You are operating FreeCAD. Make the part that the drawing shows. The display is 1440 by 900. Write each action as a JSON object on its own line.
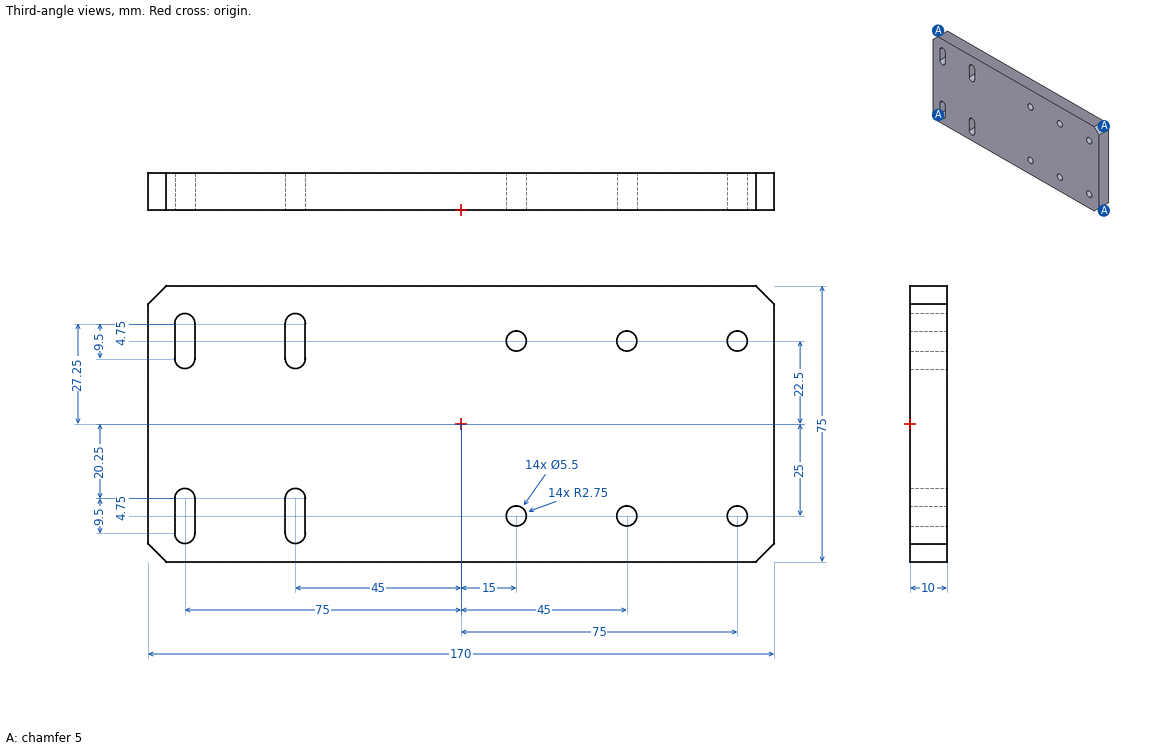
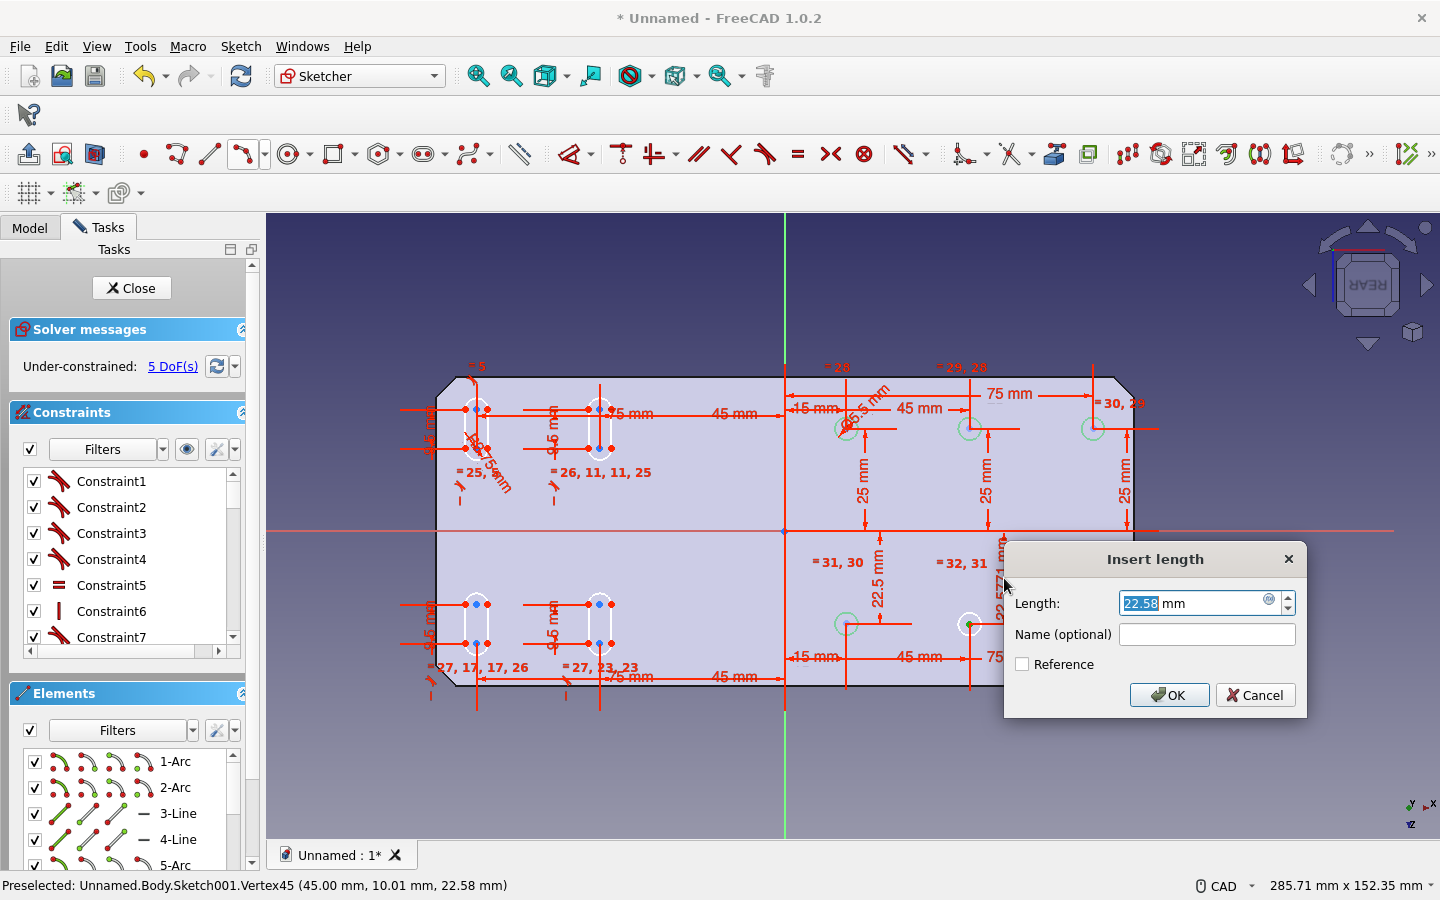
{"action": "type", "text": "22.5"}
{"action": "key", "text": "Return"}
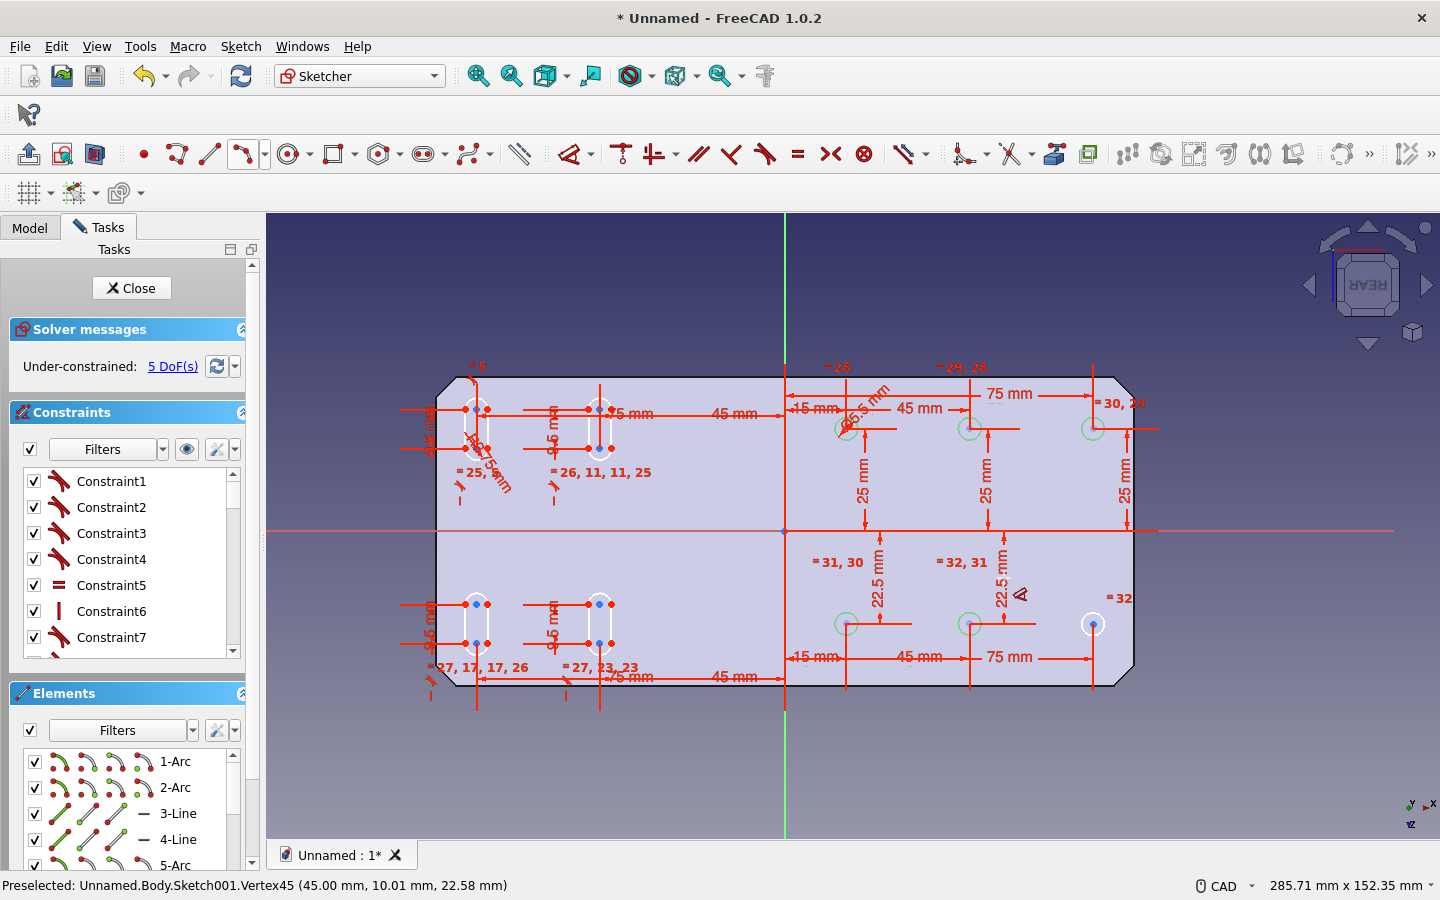
{"action": "left_click", "coordinate": [1093, 624]}
{"action": "left_click", "coordinate": [1127, 578]}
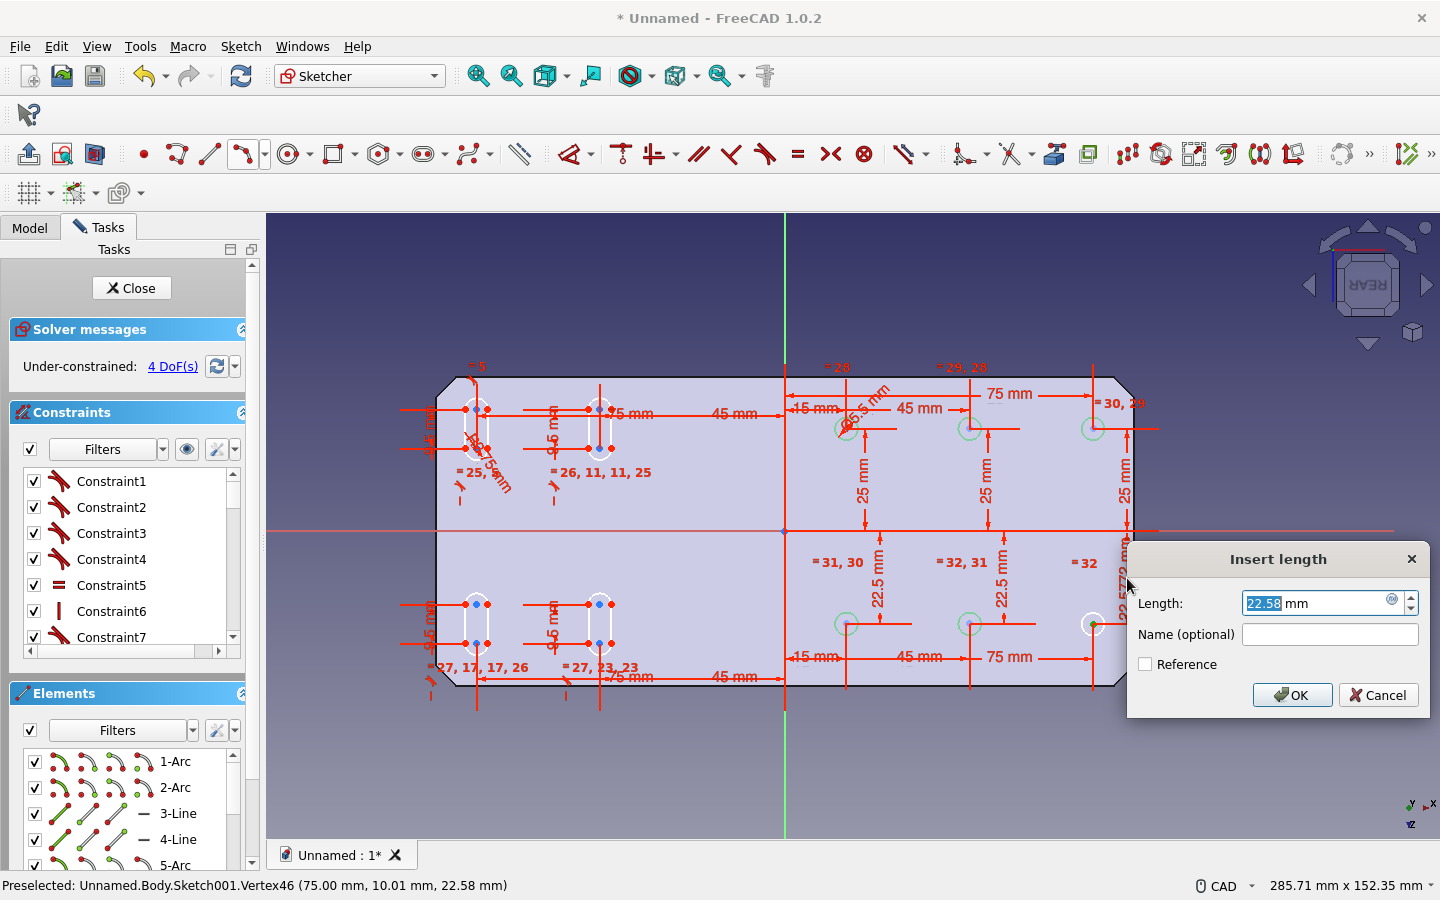
{"action": "type", "text": "22.5"}
{"action": "key", "text": "Return"}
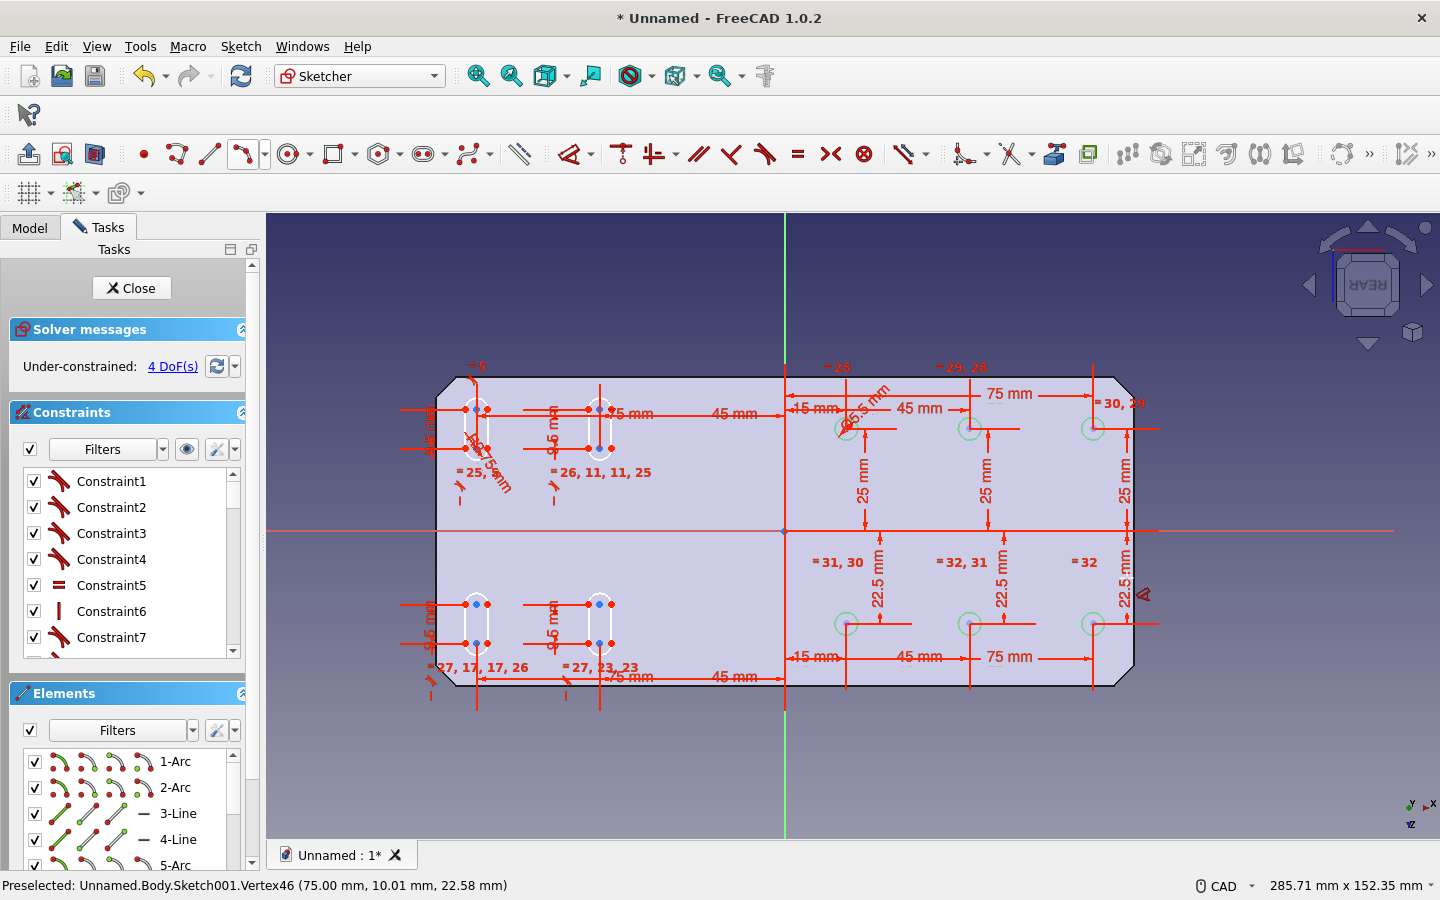
{"action": "scroll", "coordinate": [611, 449], "scroll_direction": "up", "scroll_amount": 4}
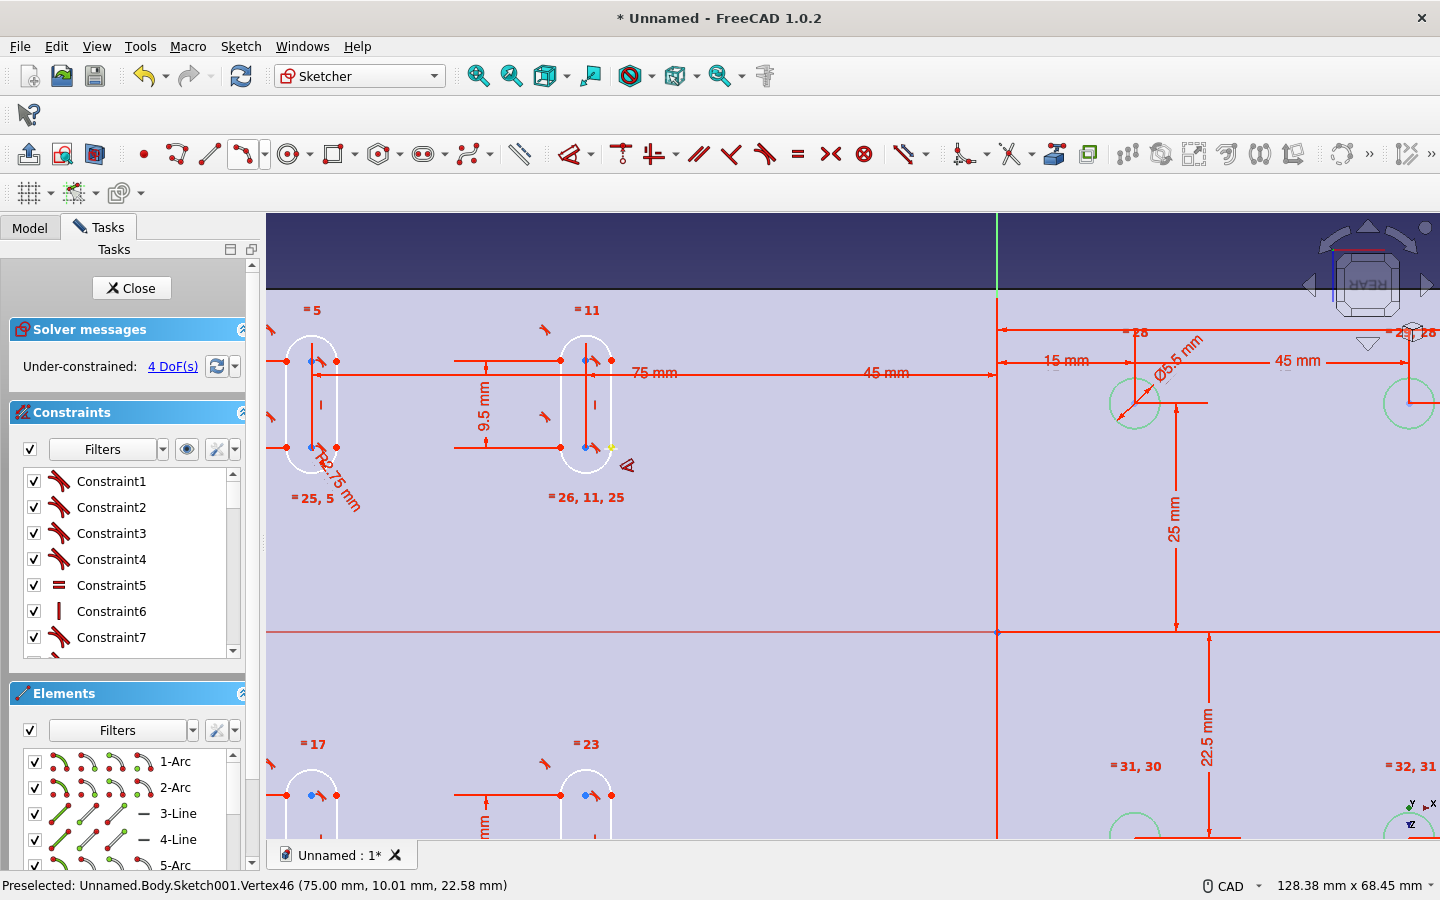
{"action": "left_click", "coordinate": [611, 448]}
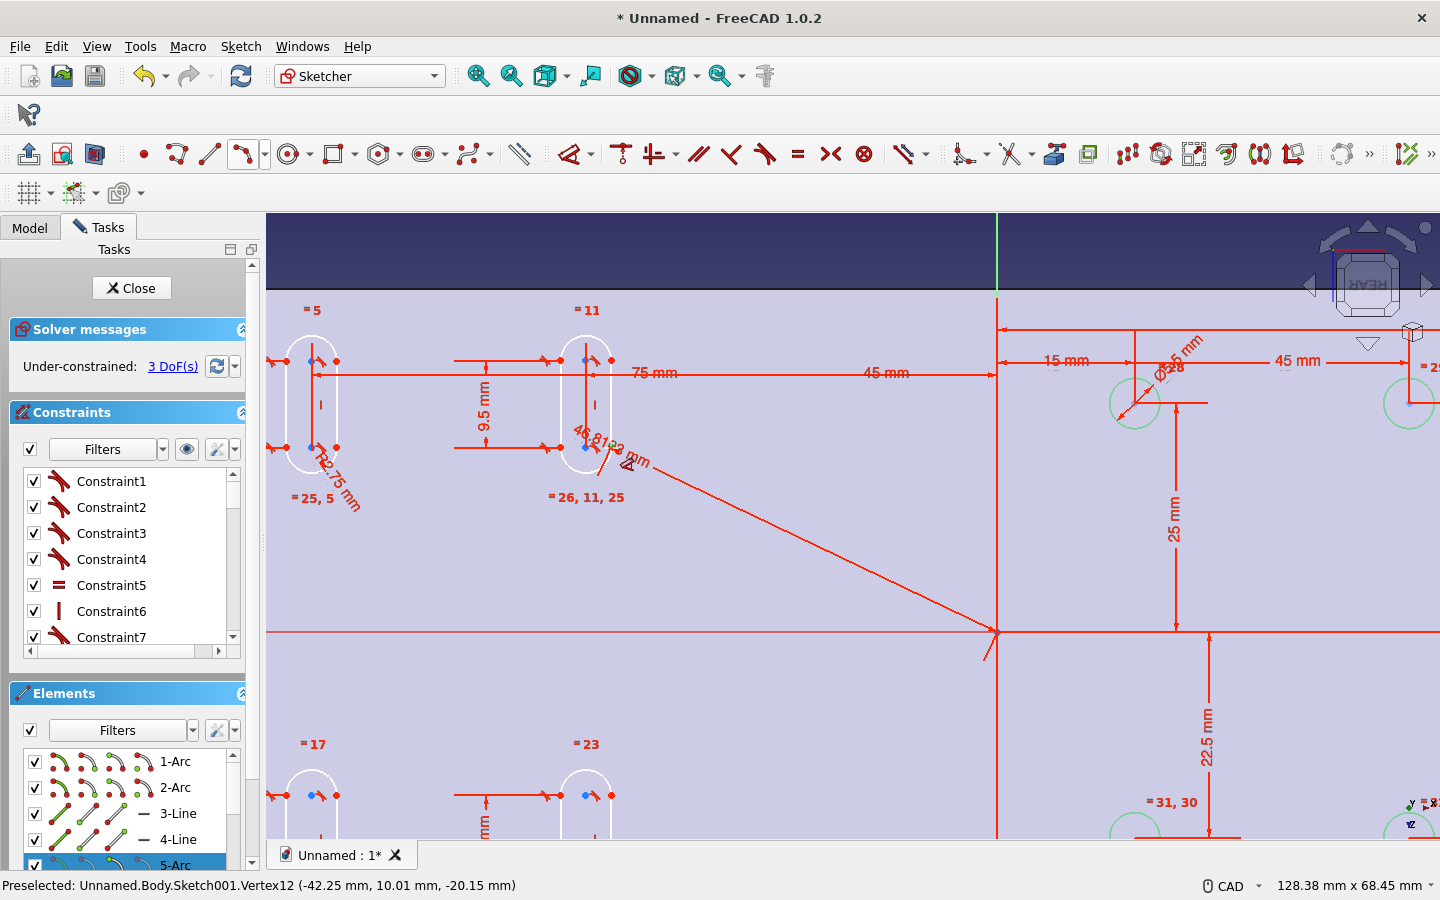
{"action": "left_click", "coordinate": [1135, 403]}
{"action": "left_click", "coordinate": [577, 426]}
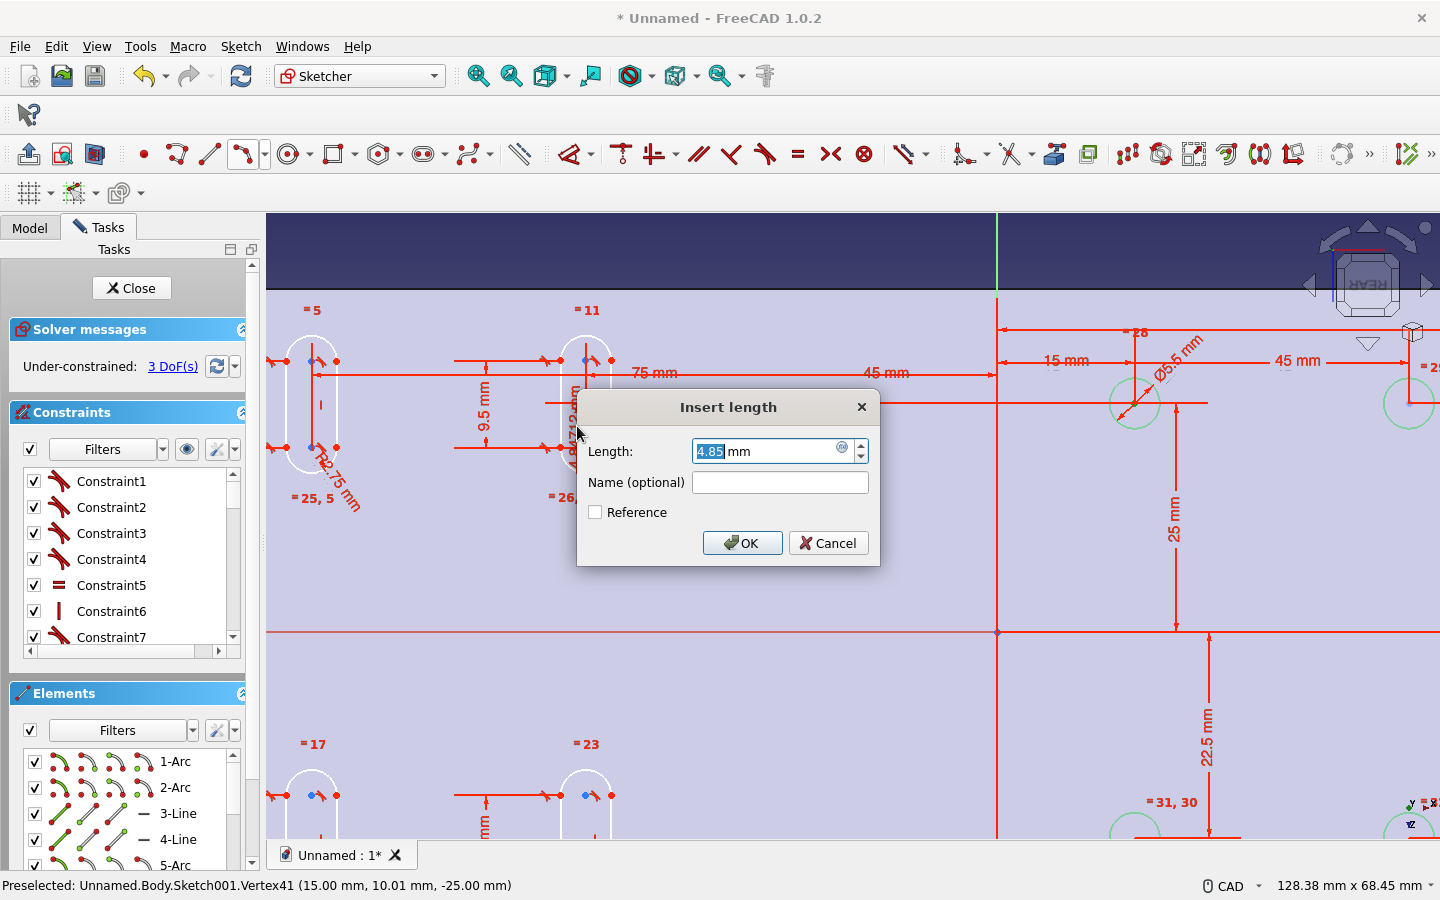
{"action": "type", "text": "4.75"}
{"action": "key", "text": "Return"}